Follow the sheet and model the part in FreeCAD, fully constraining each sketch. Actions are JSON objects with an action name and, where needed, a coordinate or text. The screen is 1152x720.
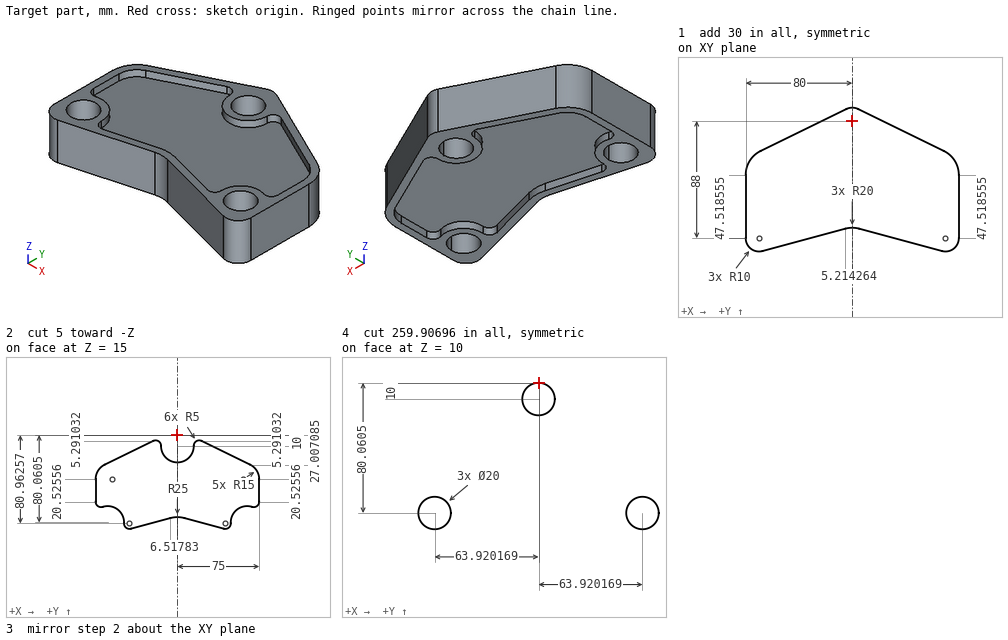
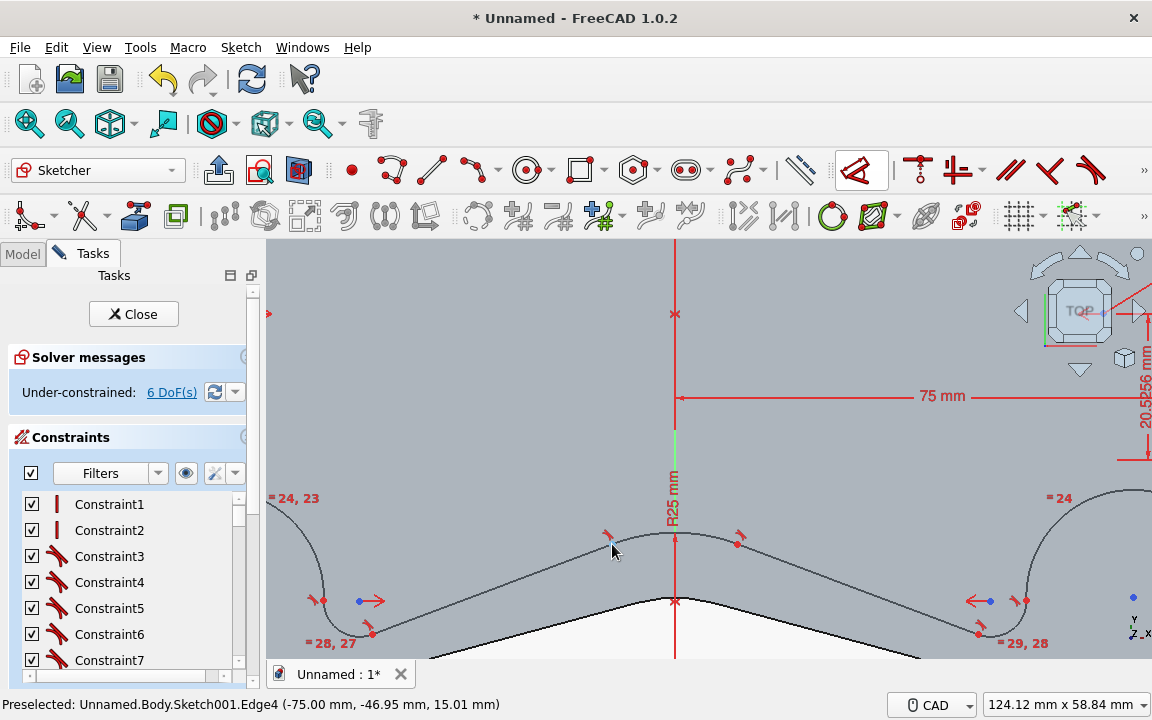
{"action": "left_click", "coordinate": [612, 544]}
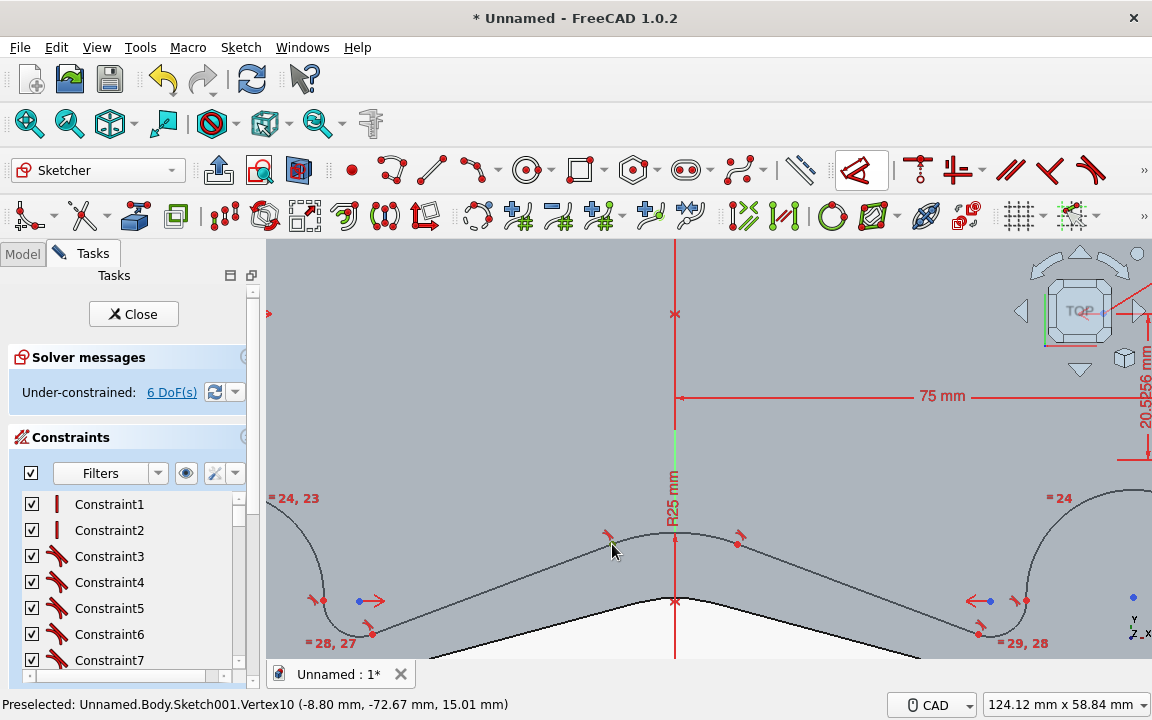
{"action": "left_click", "coordinate": [882, 170]}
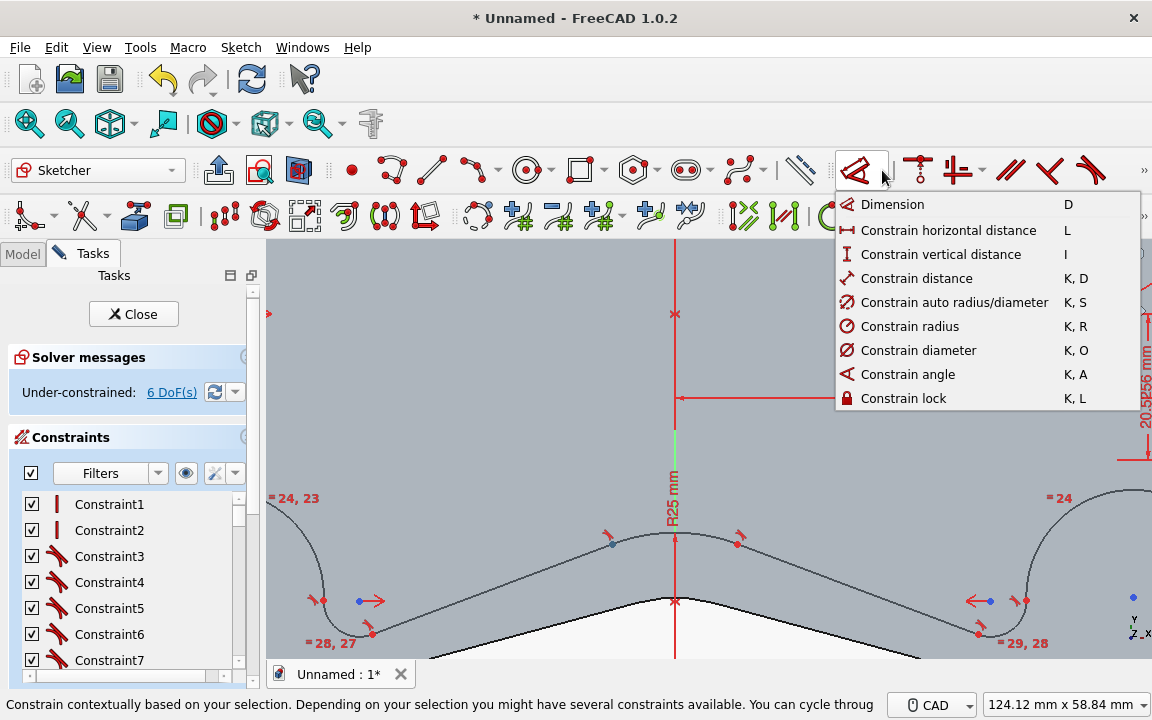
{"action": "left_click", "coordinate": [988, 230]}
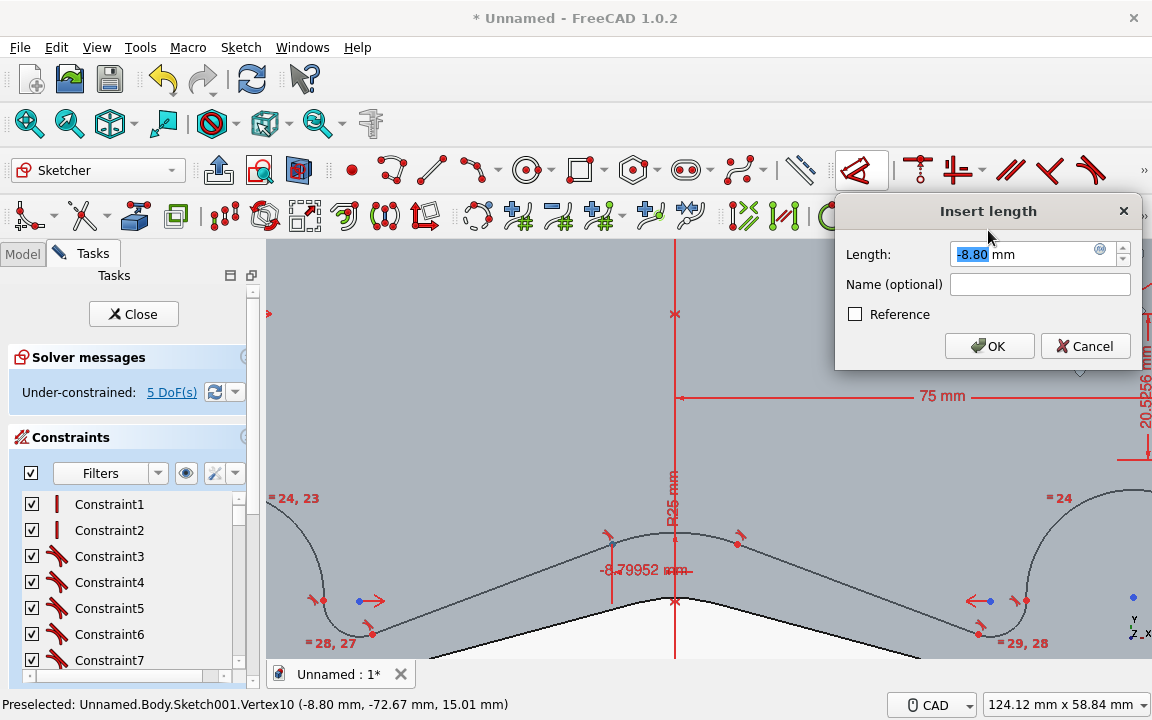
{"action": "type", "text": "-6.51783"}
{"action": "key", "text": "Return"}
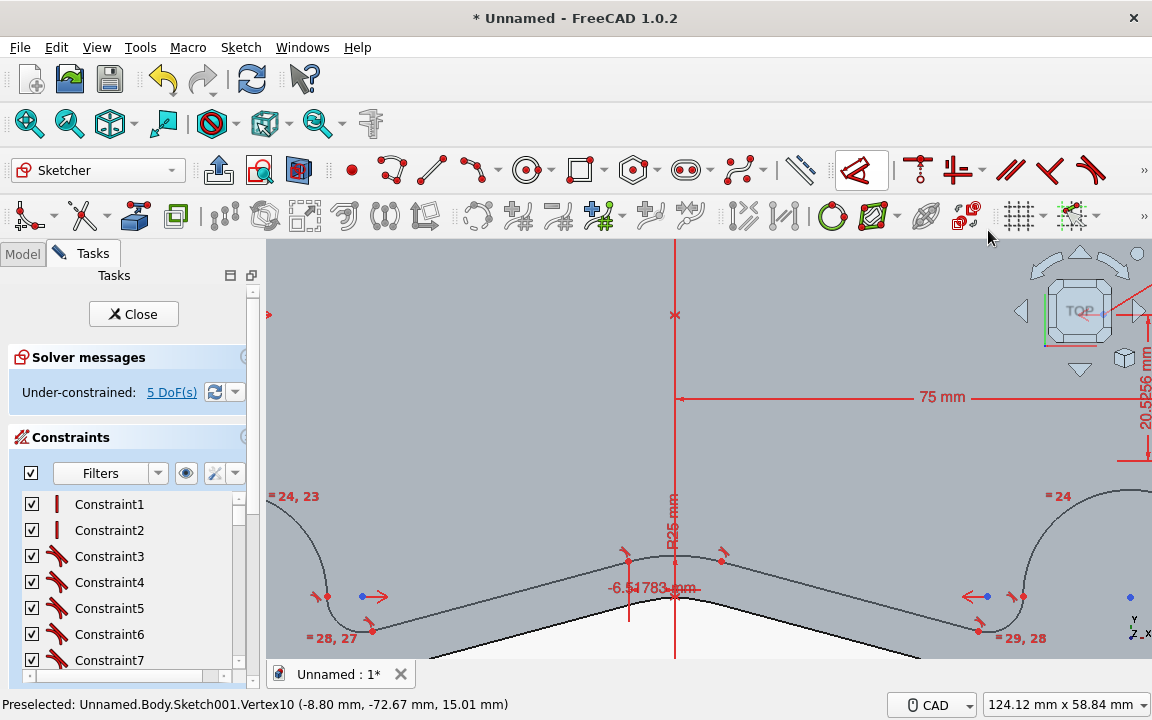
{"action": "scroll", "coordinate": [612, 545], "scroll_direction": "down", "scroll_amount": 4}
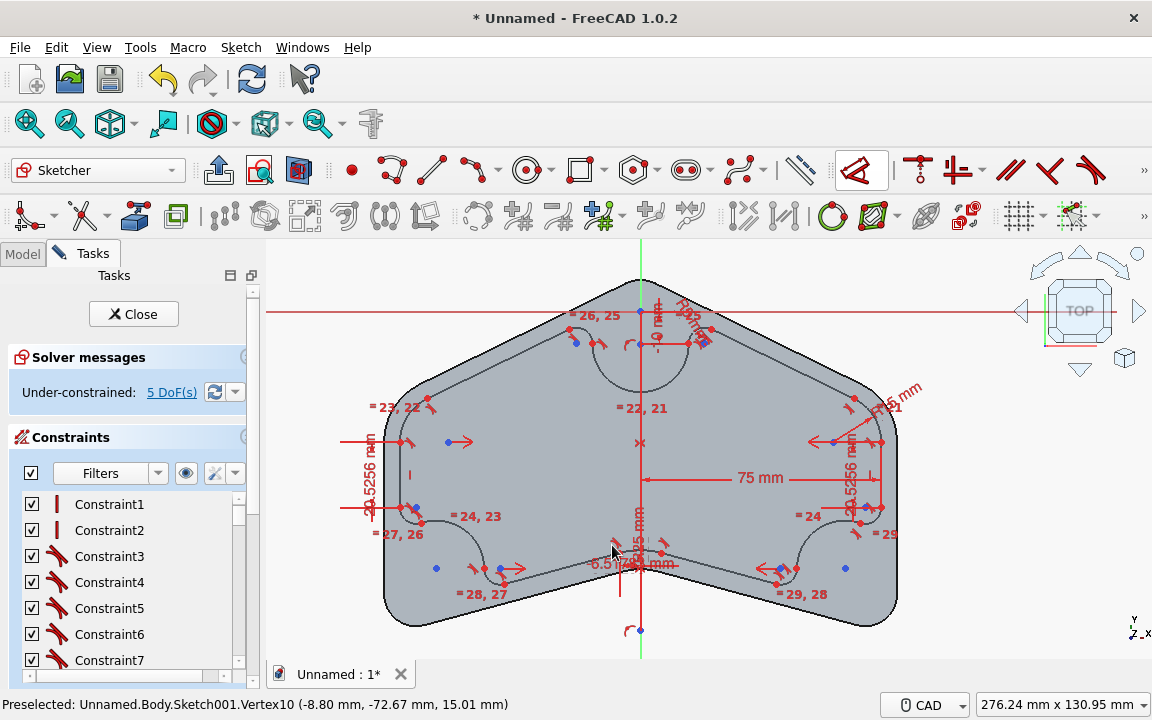
{"action": "left_click", "coordinate": [436, 569]}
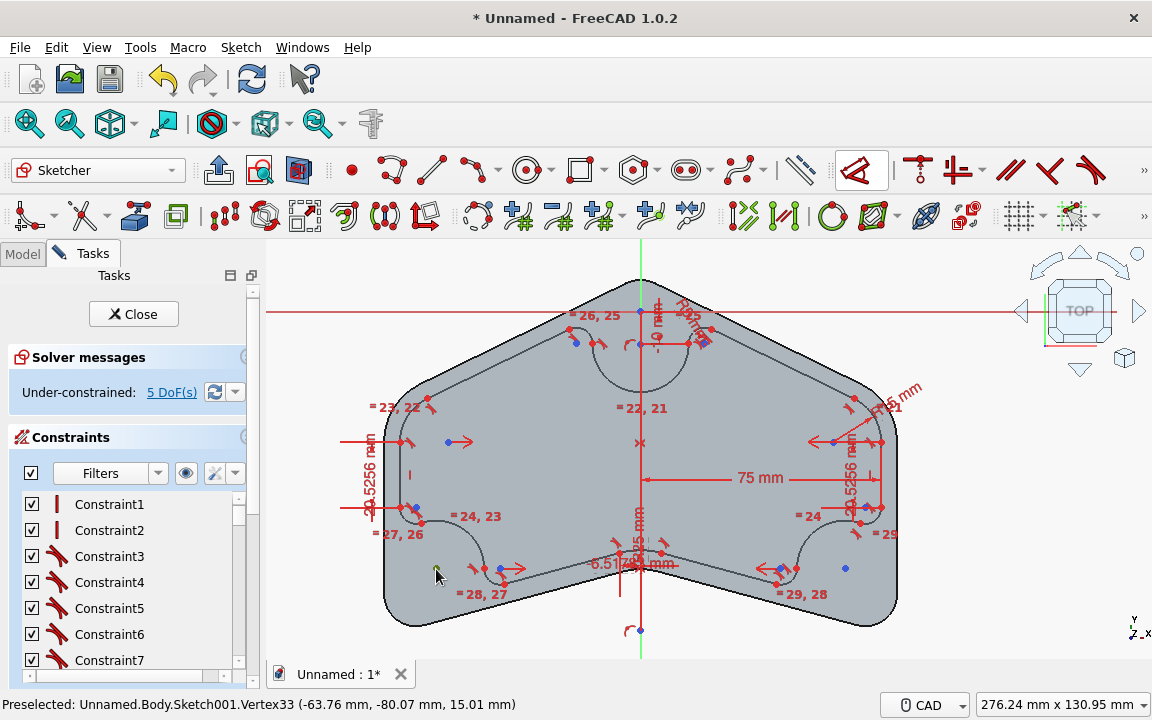
{"action": "left_click", "coordinate": [882, 170]}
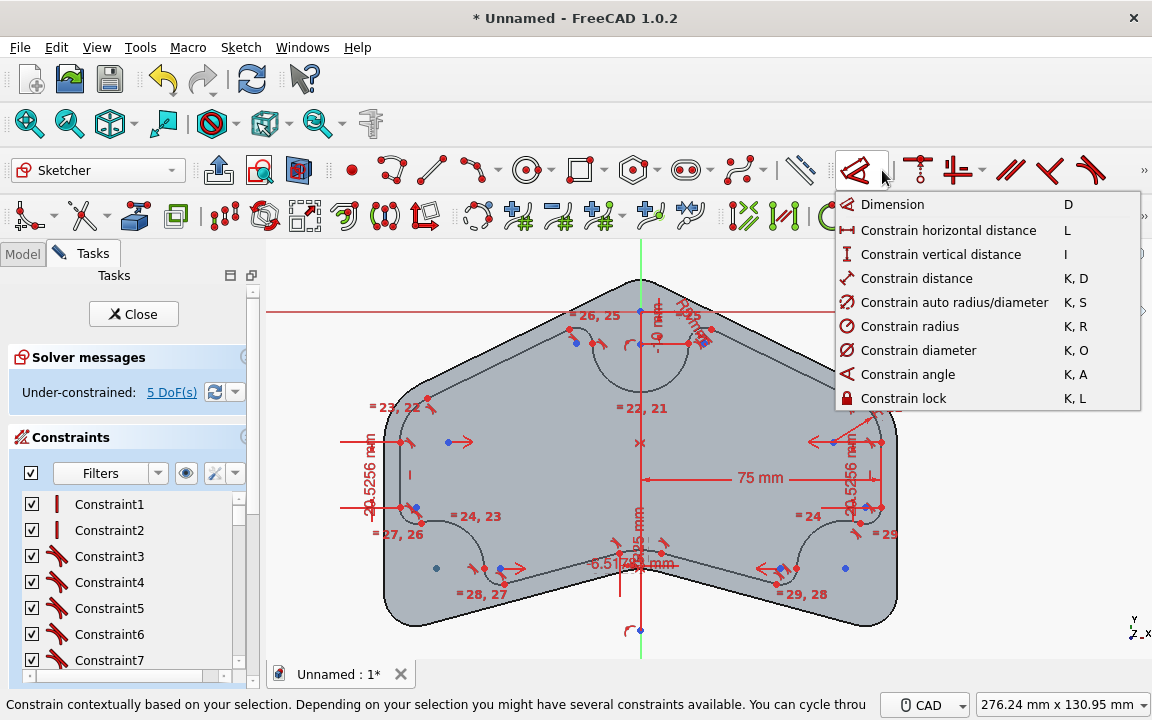
{"action": "left_click", "coordinate": [988, 254]}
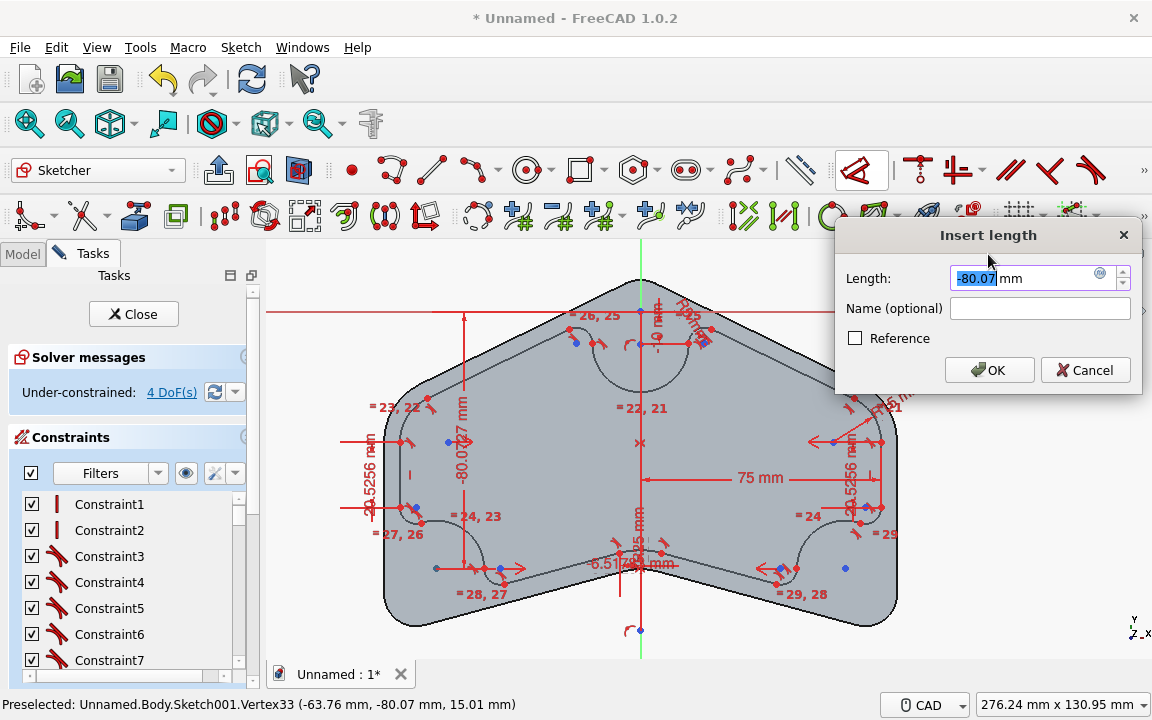
{"action": "type", "text": "-80.0605"}
{"action": "key", "text": "Return"}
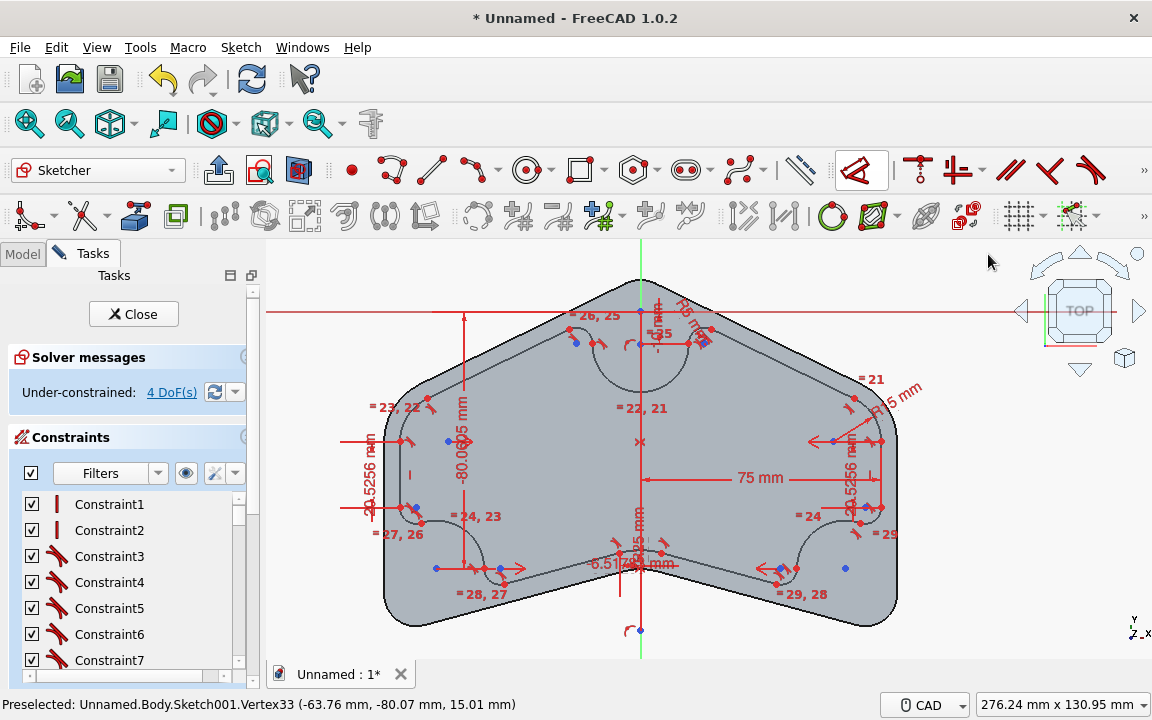
{"action": "scroll", "coordinate": [712, 329], "scroll_direction": "up", "scroll_amount": 5}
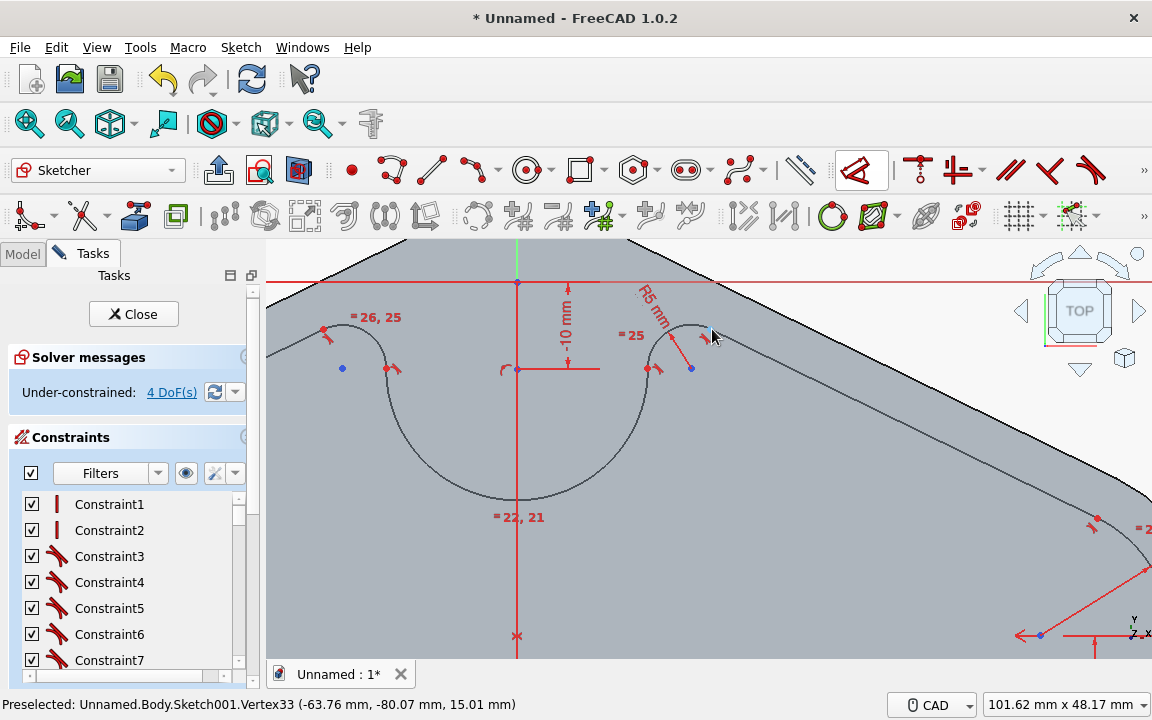
{"action": "left_click", "coordinate": [711, 329]}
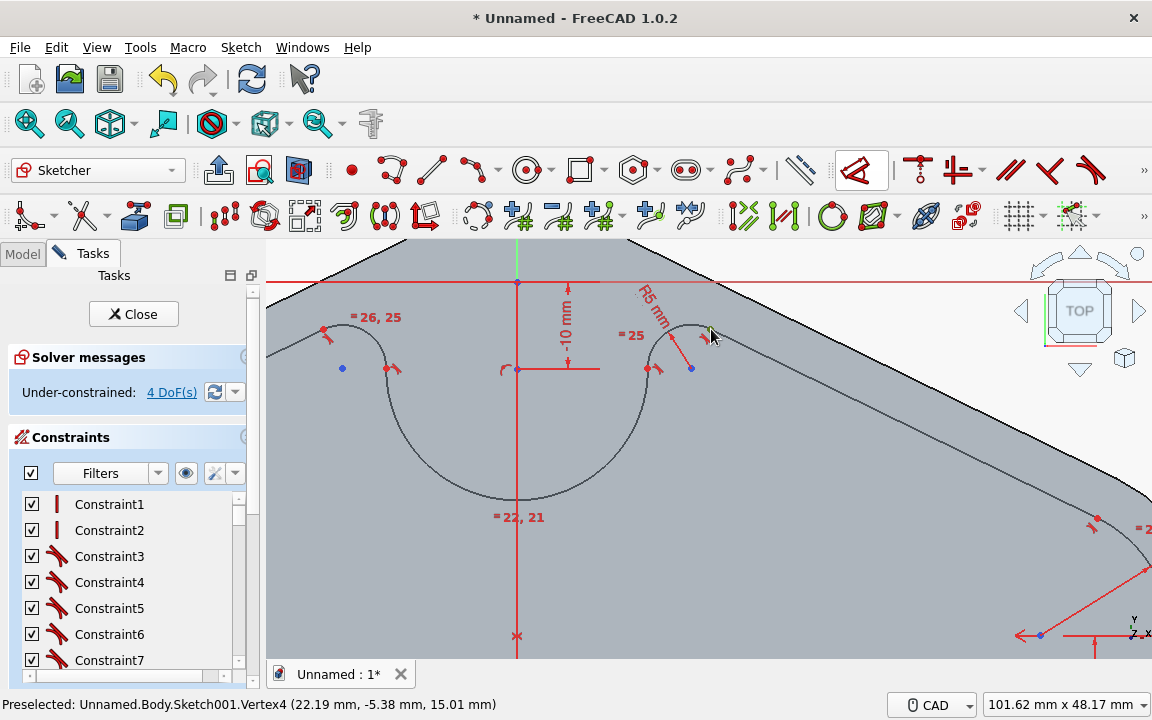
{"action": "left_click", "coordinate": [882, 170]}